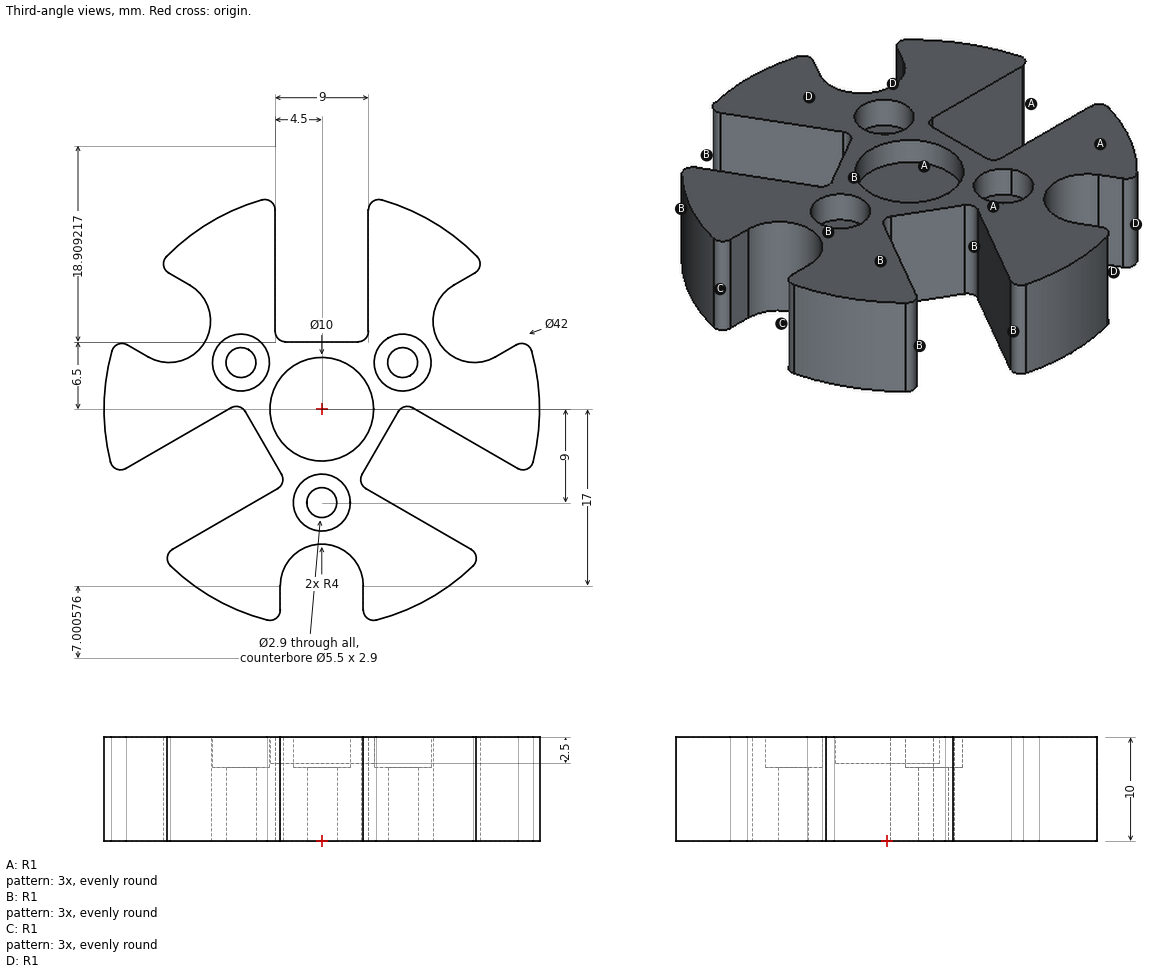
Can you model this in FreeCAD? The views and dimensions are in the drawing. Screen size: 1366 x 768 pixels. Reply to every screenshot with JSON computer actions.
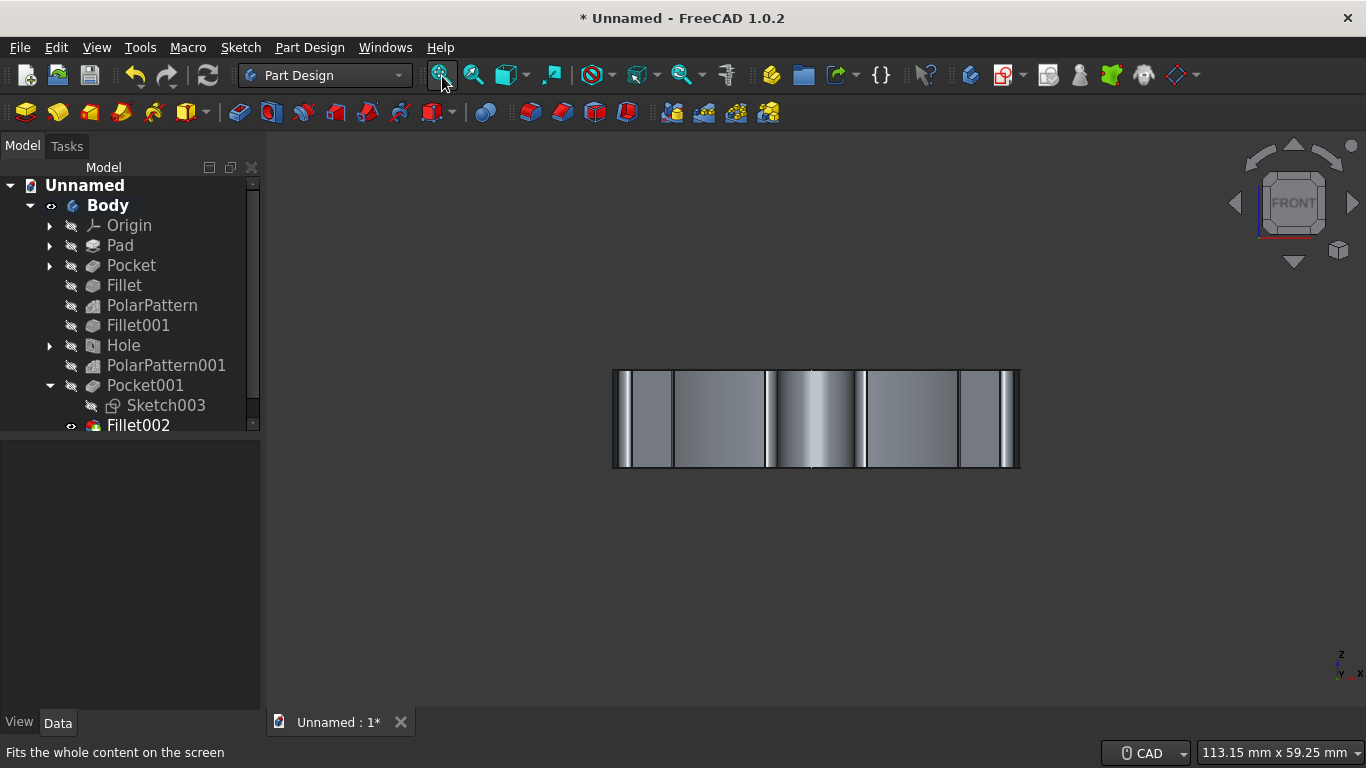
{"action": "left_click", "coordinate": [116, 386]}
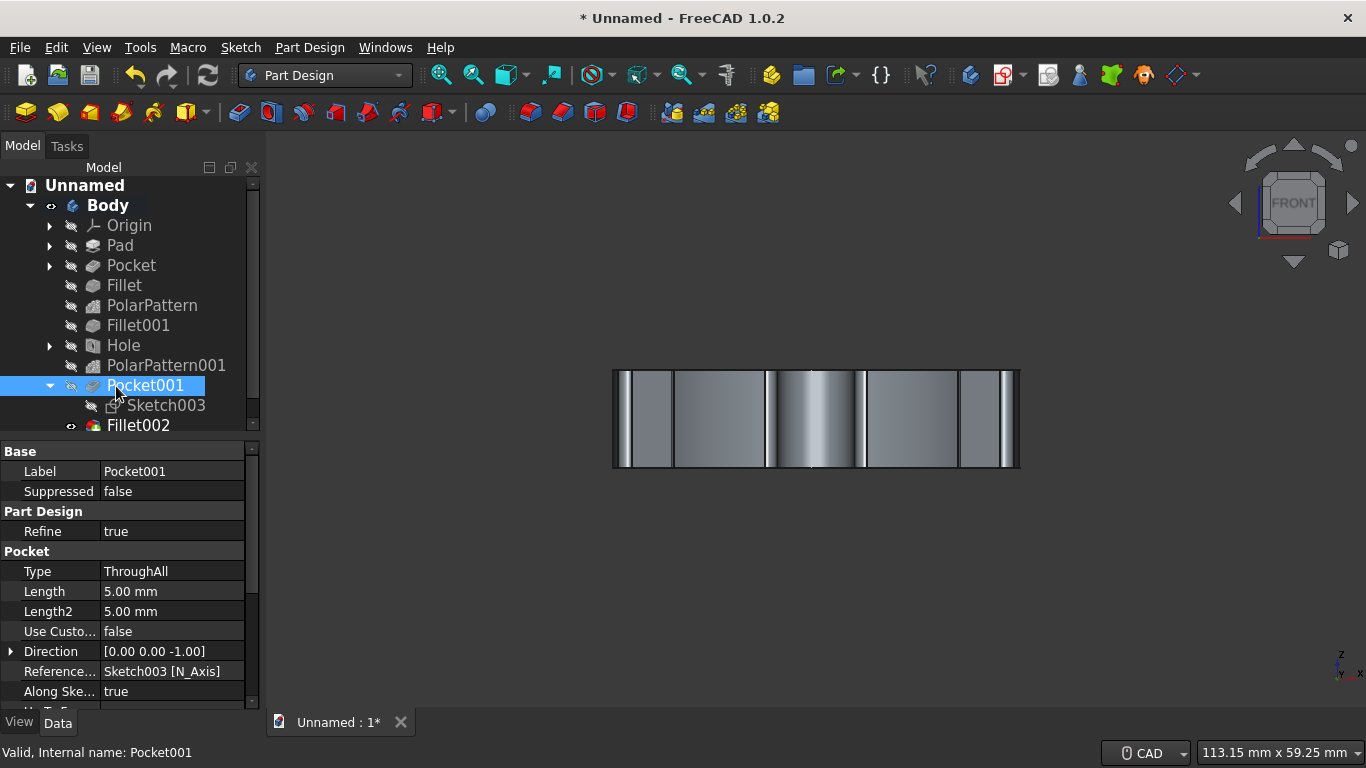
{"action": "left_click", "coordinate": [736, 112]}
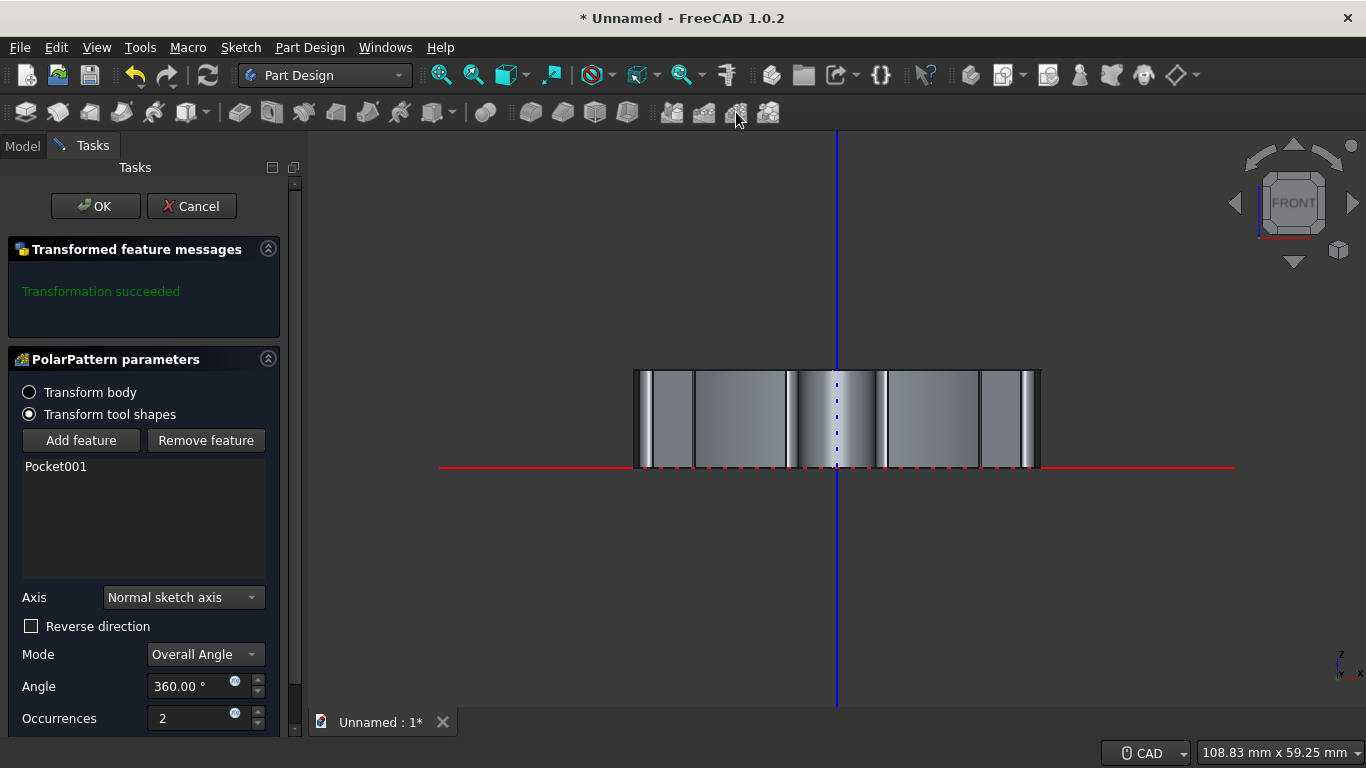
{"action": "left_click", "coordinate": [184, 598]}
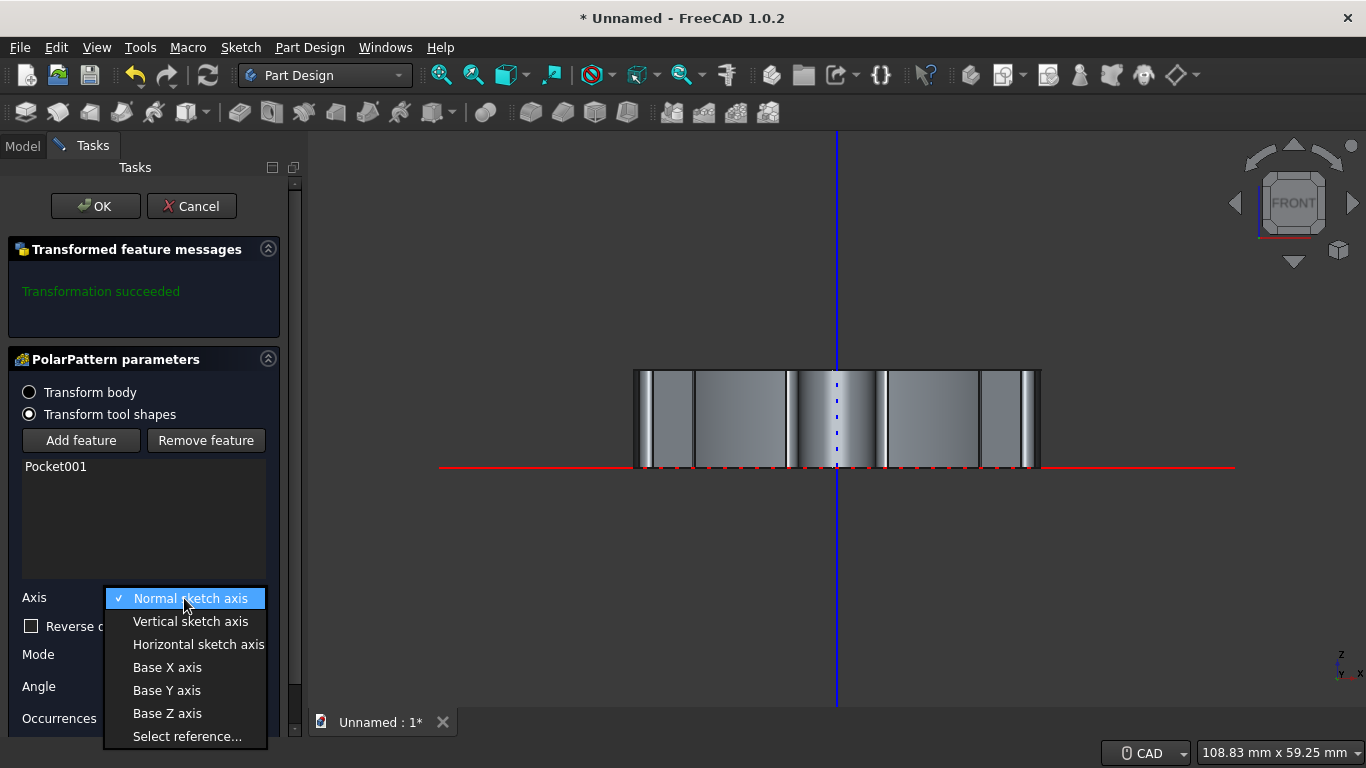
{"action": "left_click", "coordinate": [184, 714]}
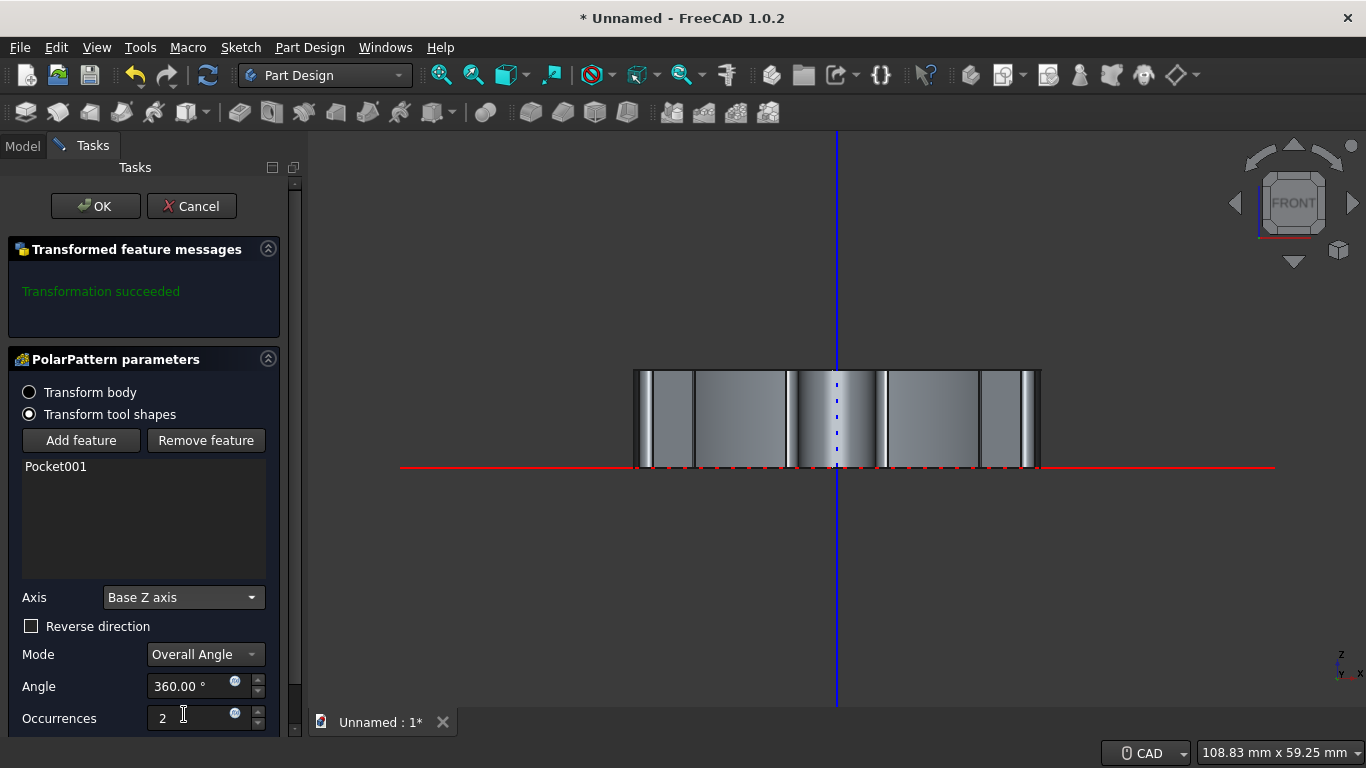
{"action": "triple_click", "coordinate": [198, 718]}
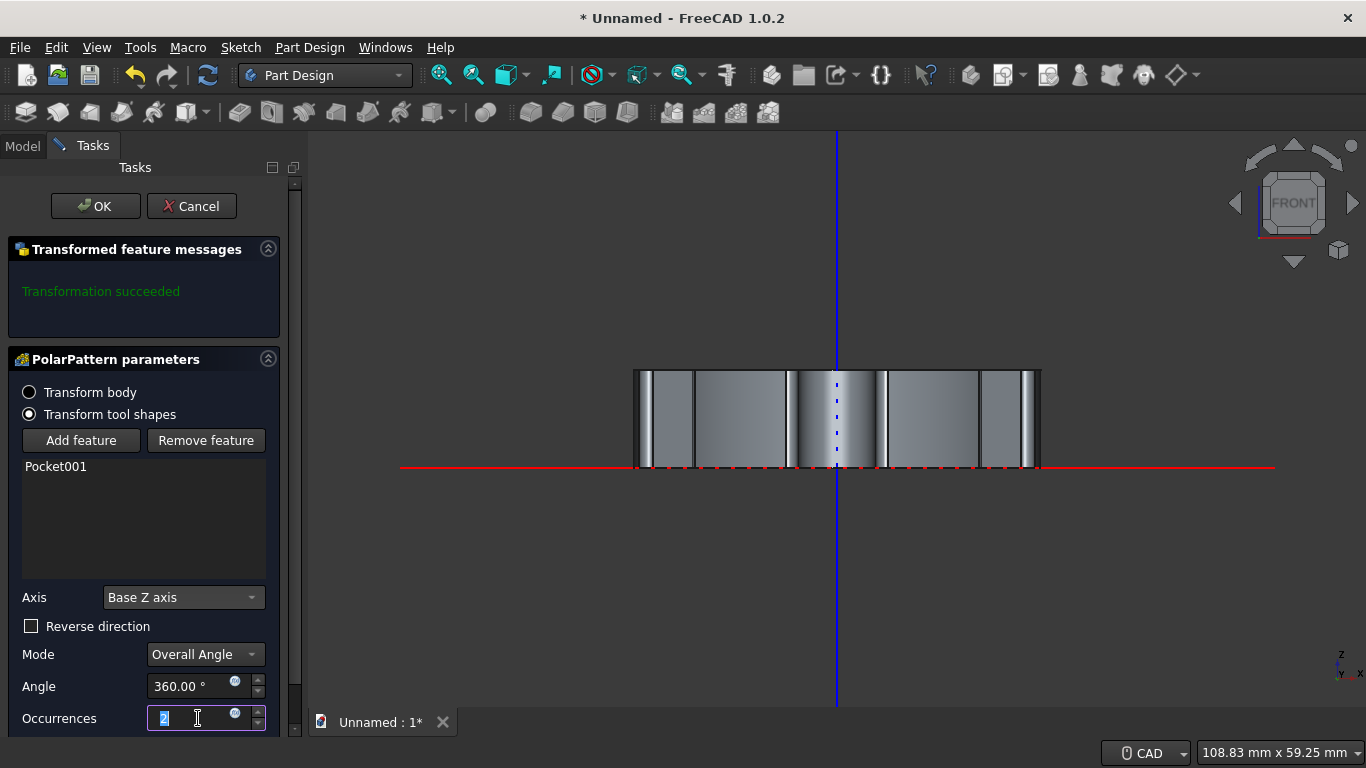
{"action": "type", "text": "3"}
{"action": "key", "text": "Tab"}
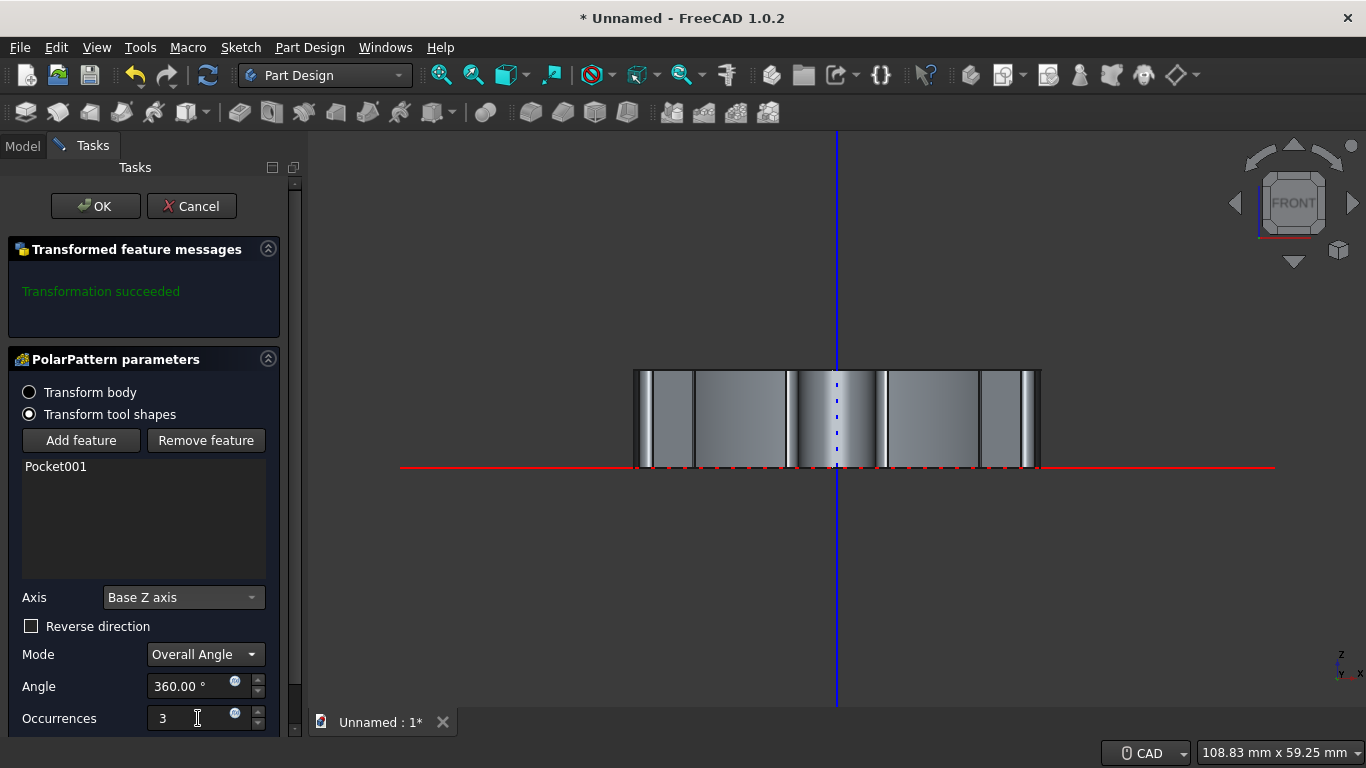
{"action": "left_click", "coordinate": [96, 206]}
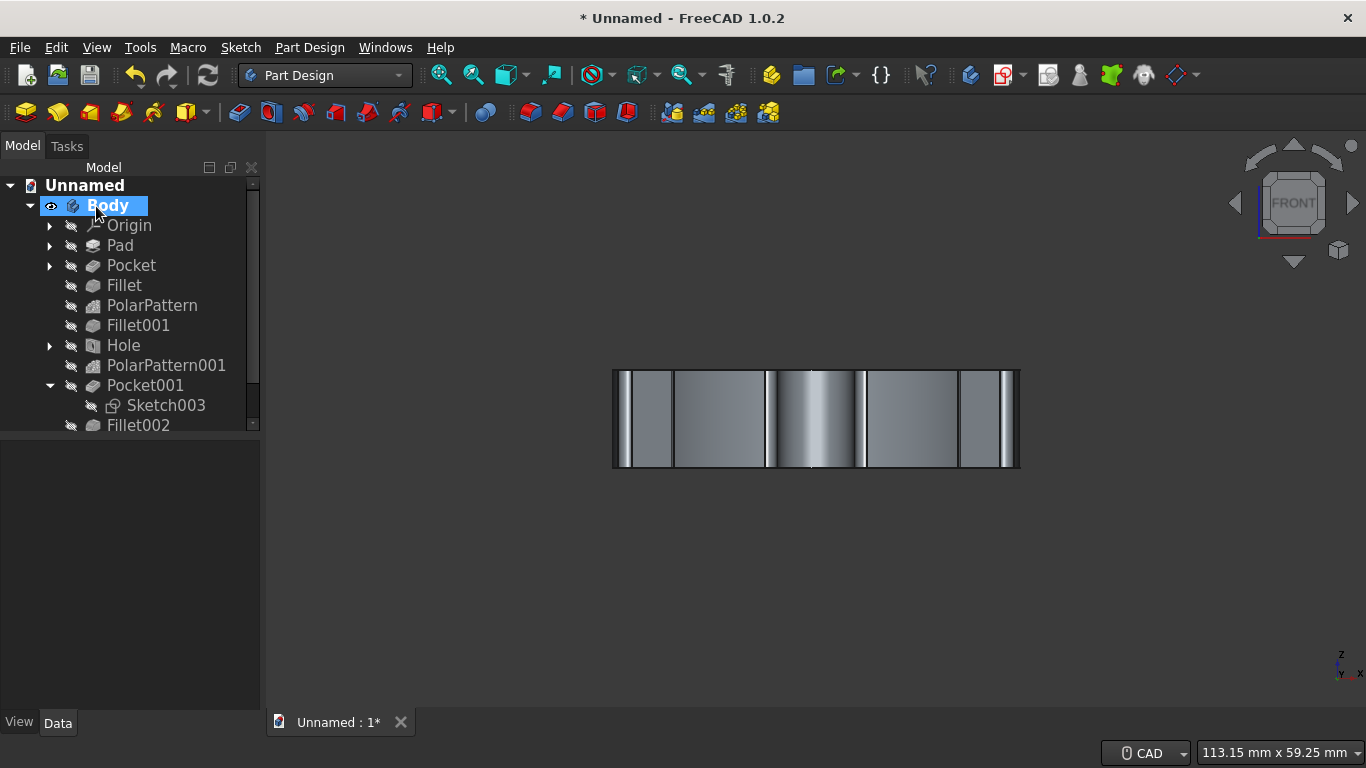
{"action": "left_click", "coordinate": [442, 76]}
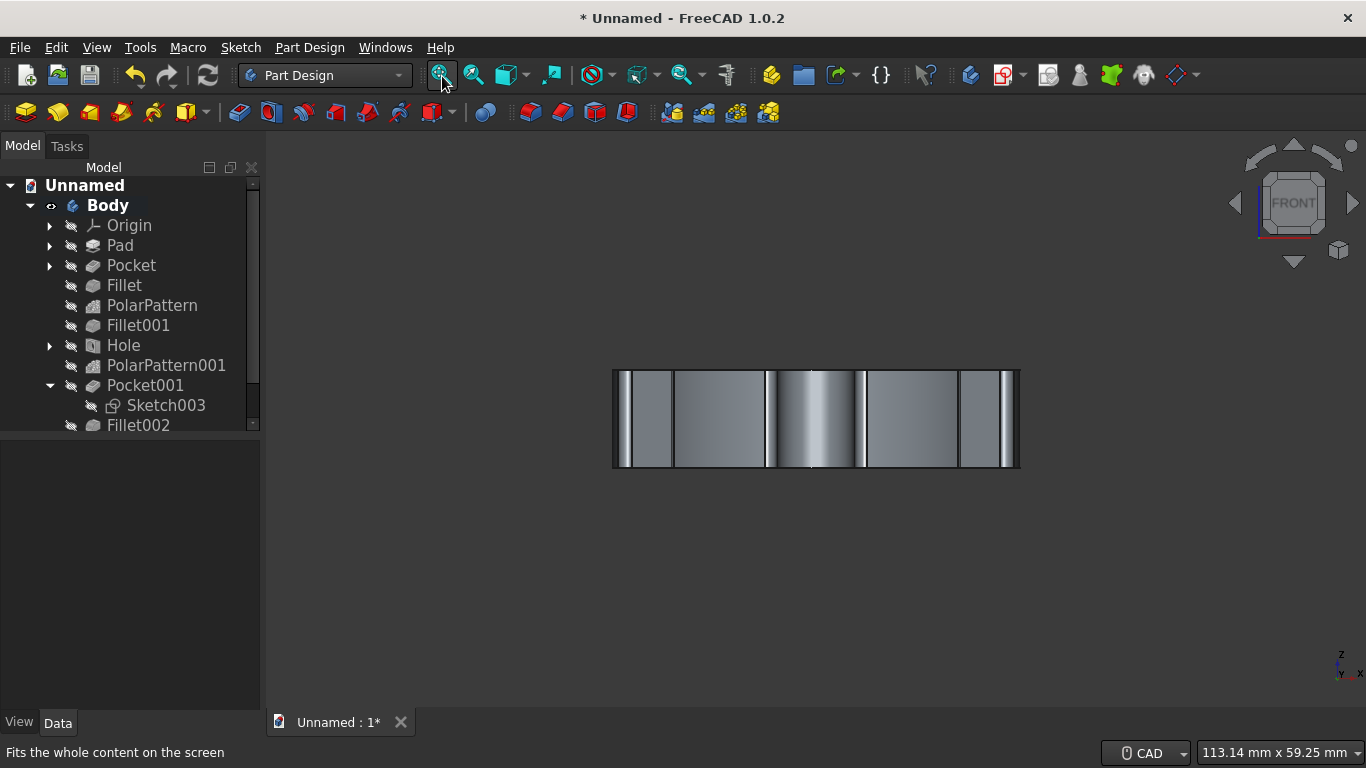
{"action": "key", "text": "0"}